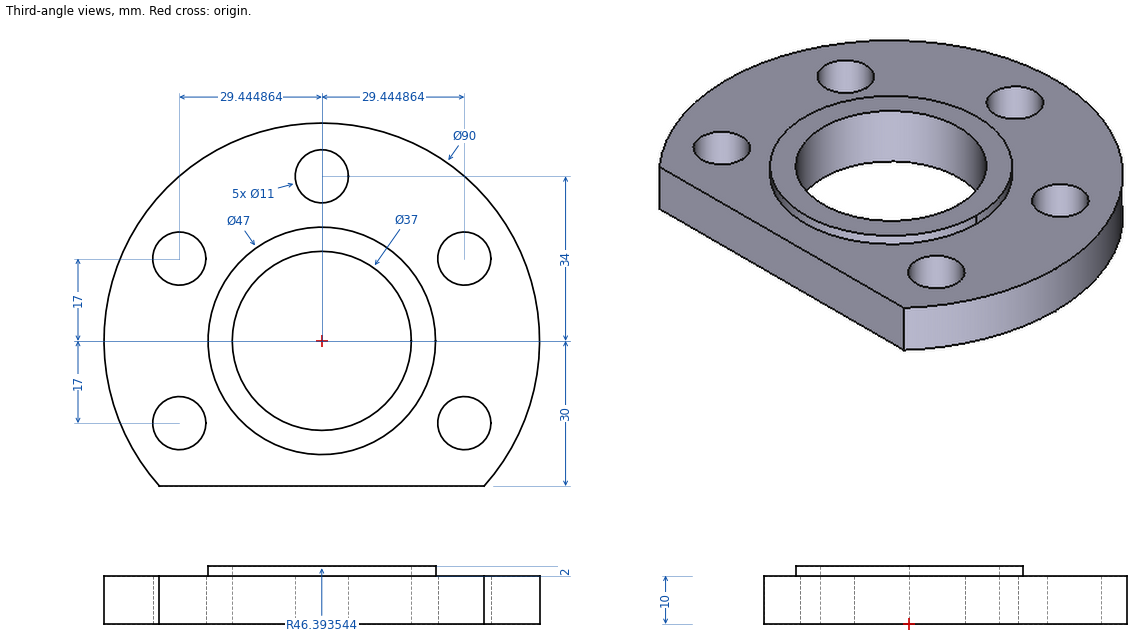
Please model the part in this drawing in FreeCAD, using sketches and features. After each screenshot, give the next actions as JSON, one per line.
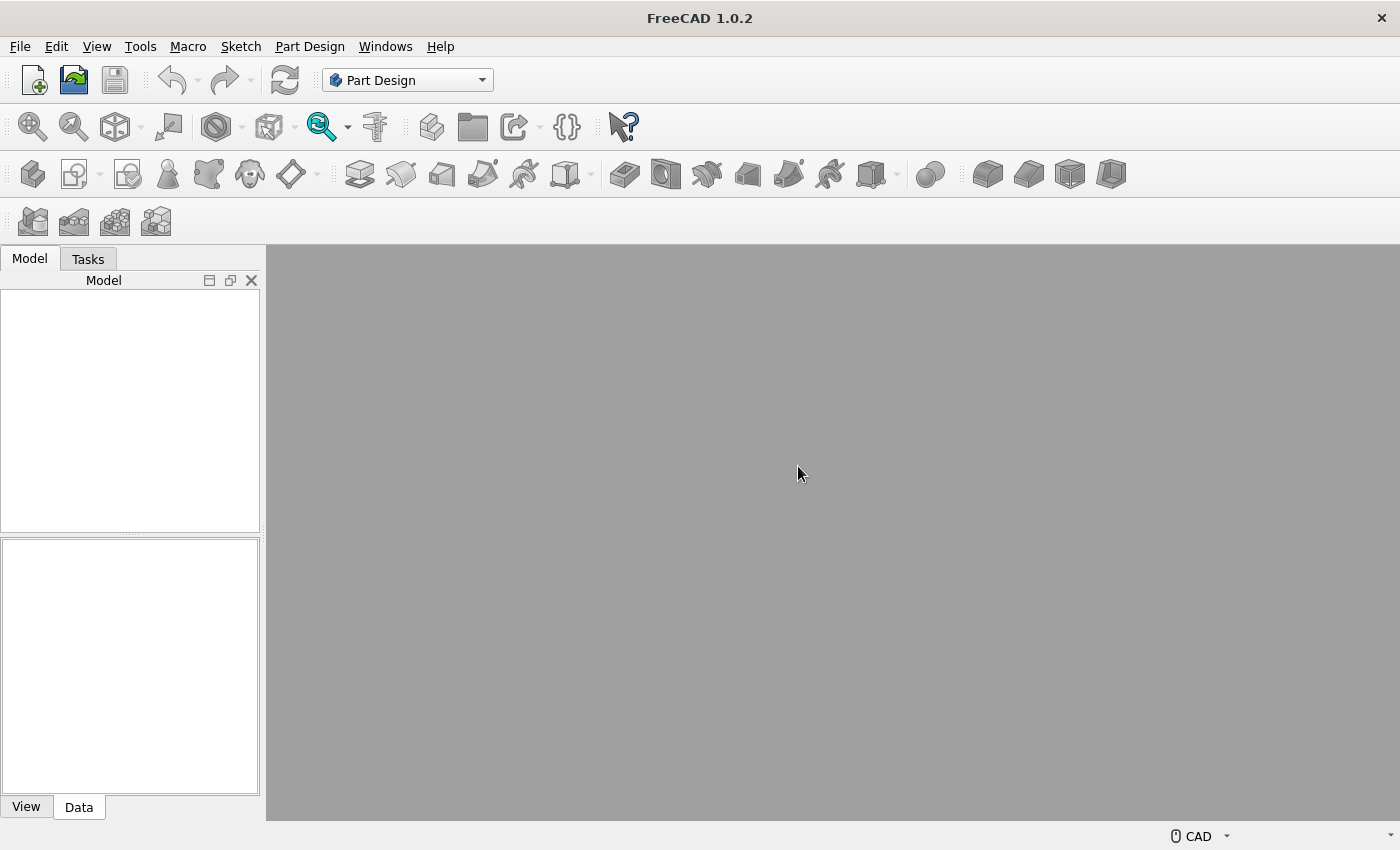
{"action": "left_click", "coordinate": [33, 80]}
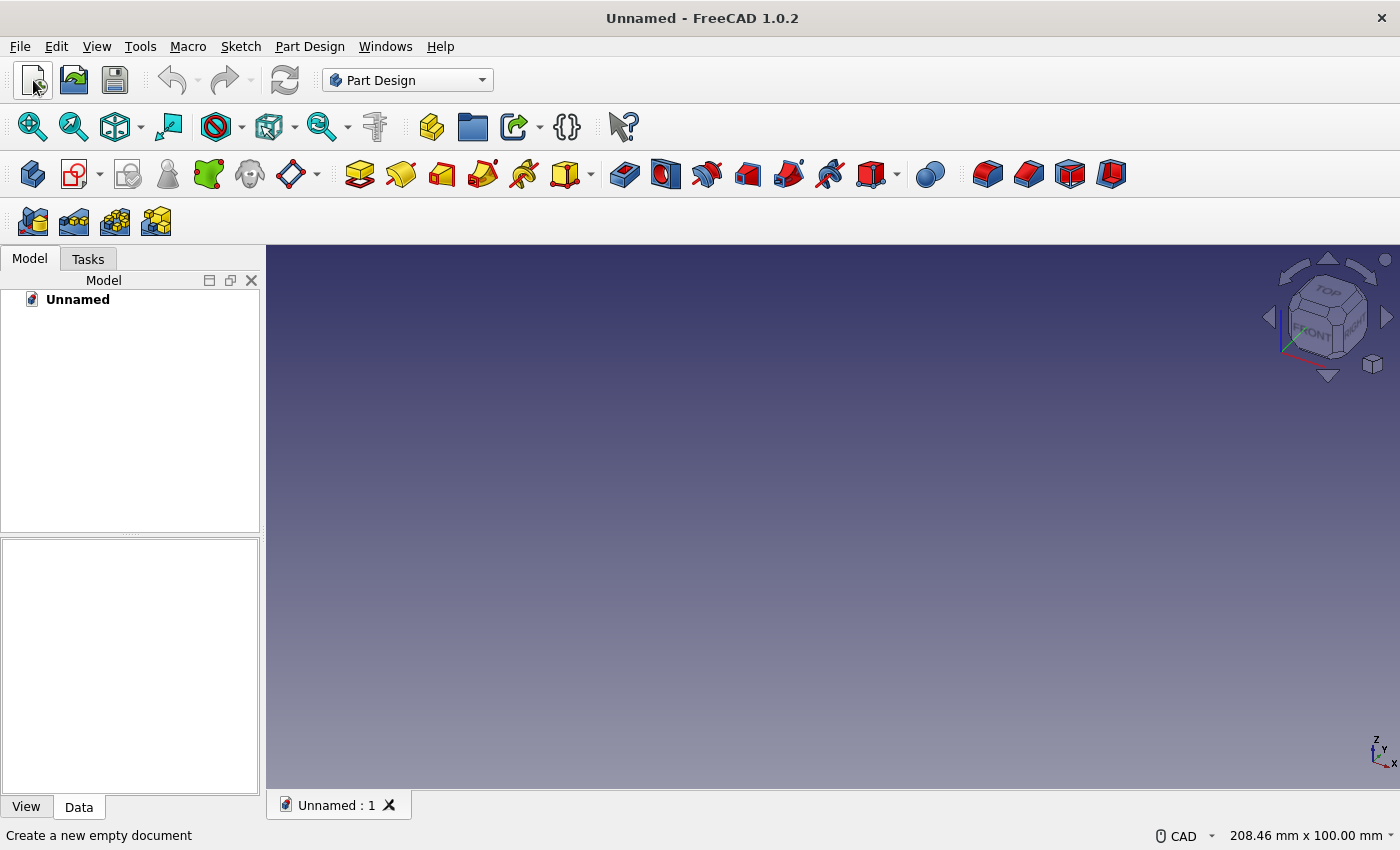
{"action": "left_click", "coordinate": [74, 174]}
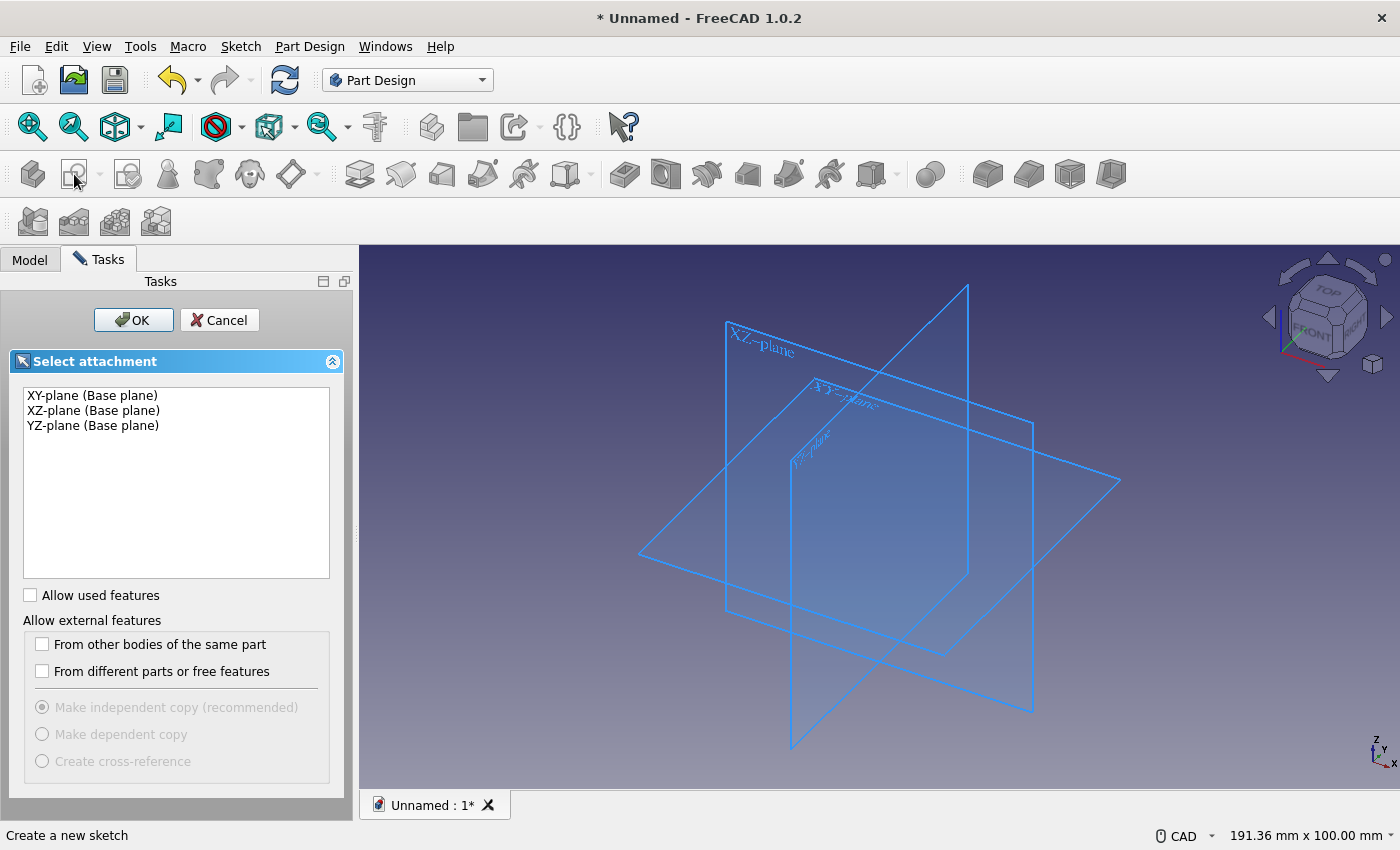
{"action": "left_click", "coordinate": [84, 396]}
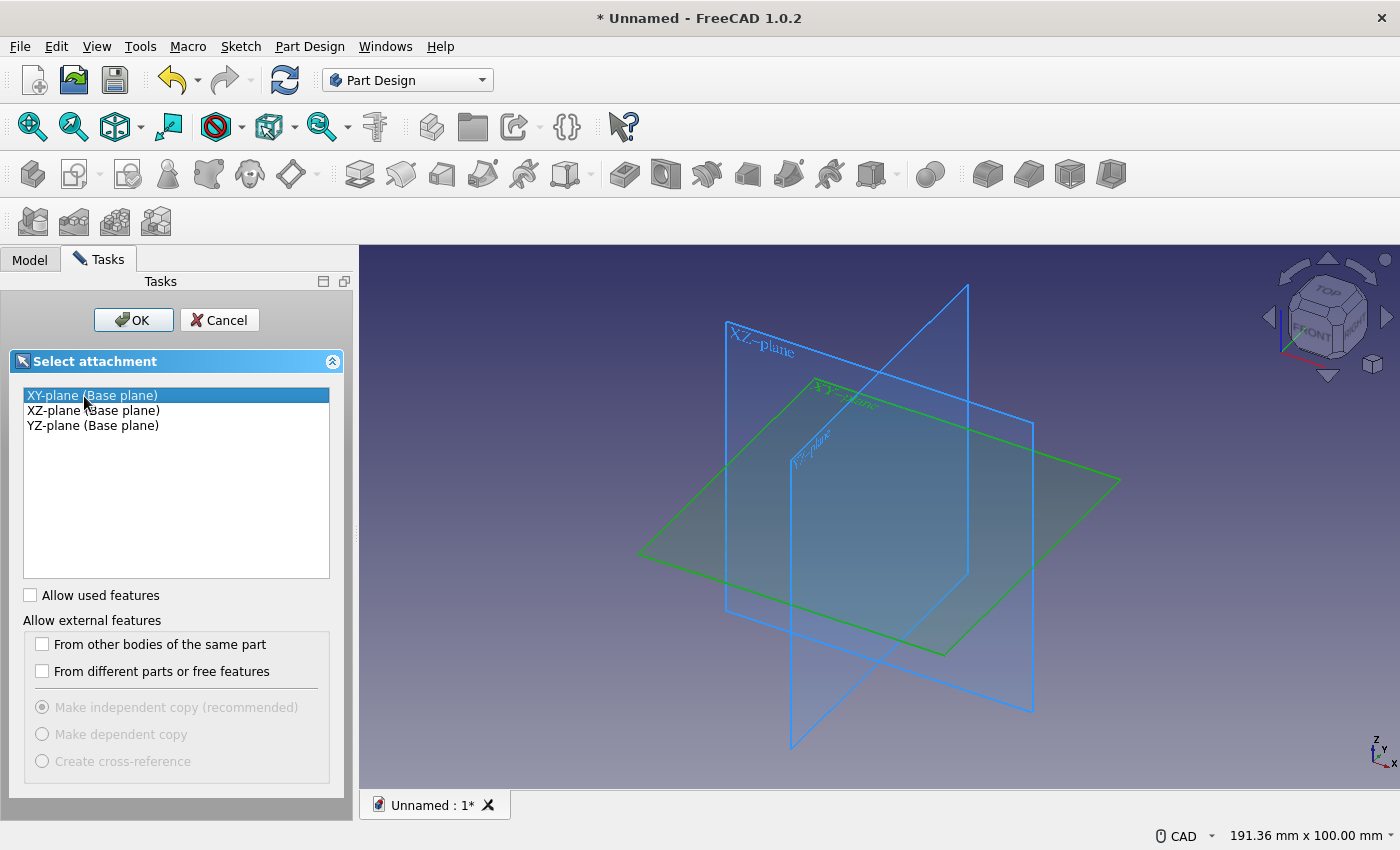
{"action": "left_click", "coordinate": [134, 320]}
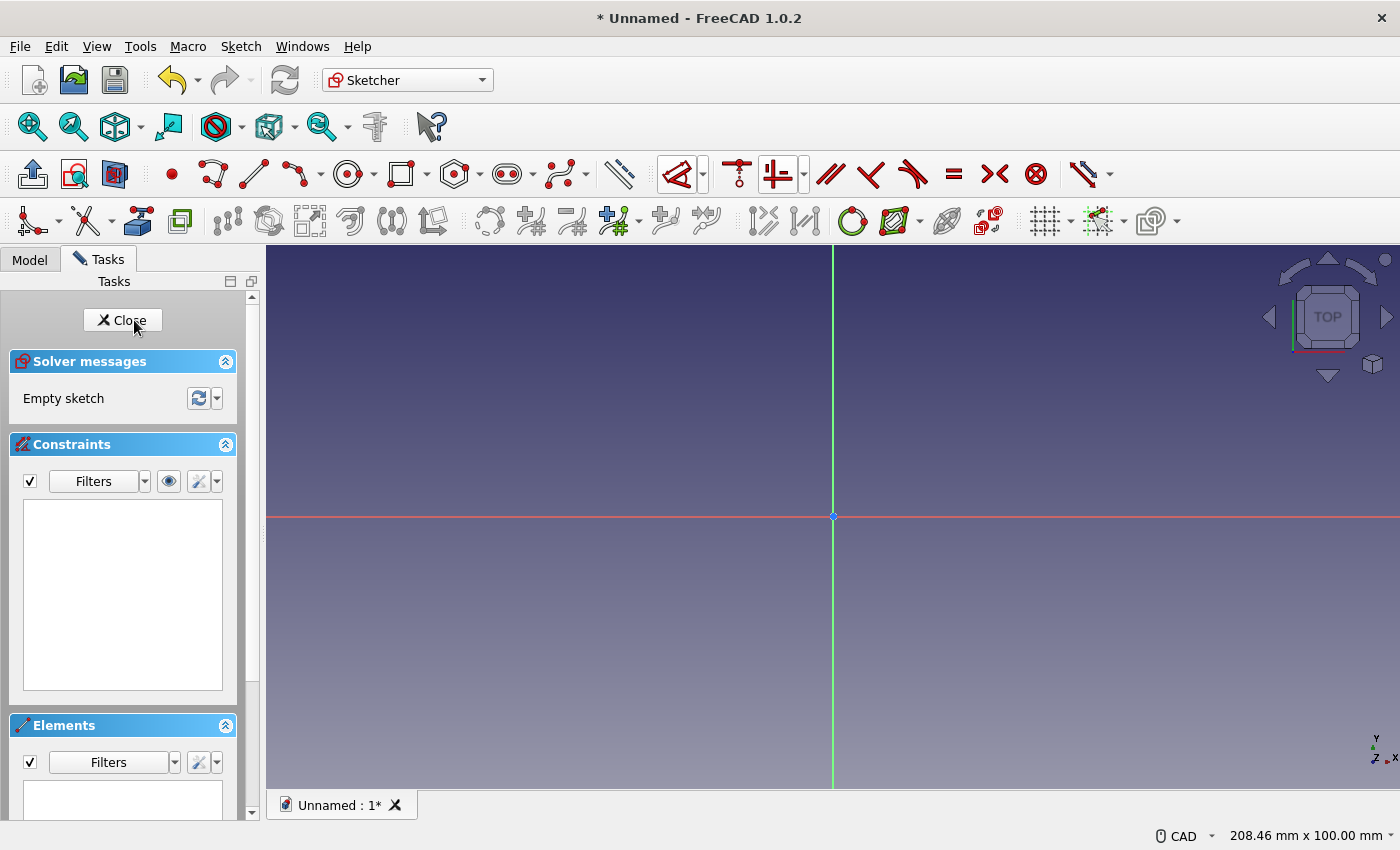
{"action": "scroll", "coordinate": [625, 517], "scroll_direction": "down", "scroll_amount": 2}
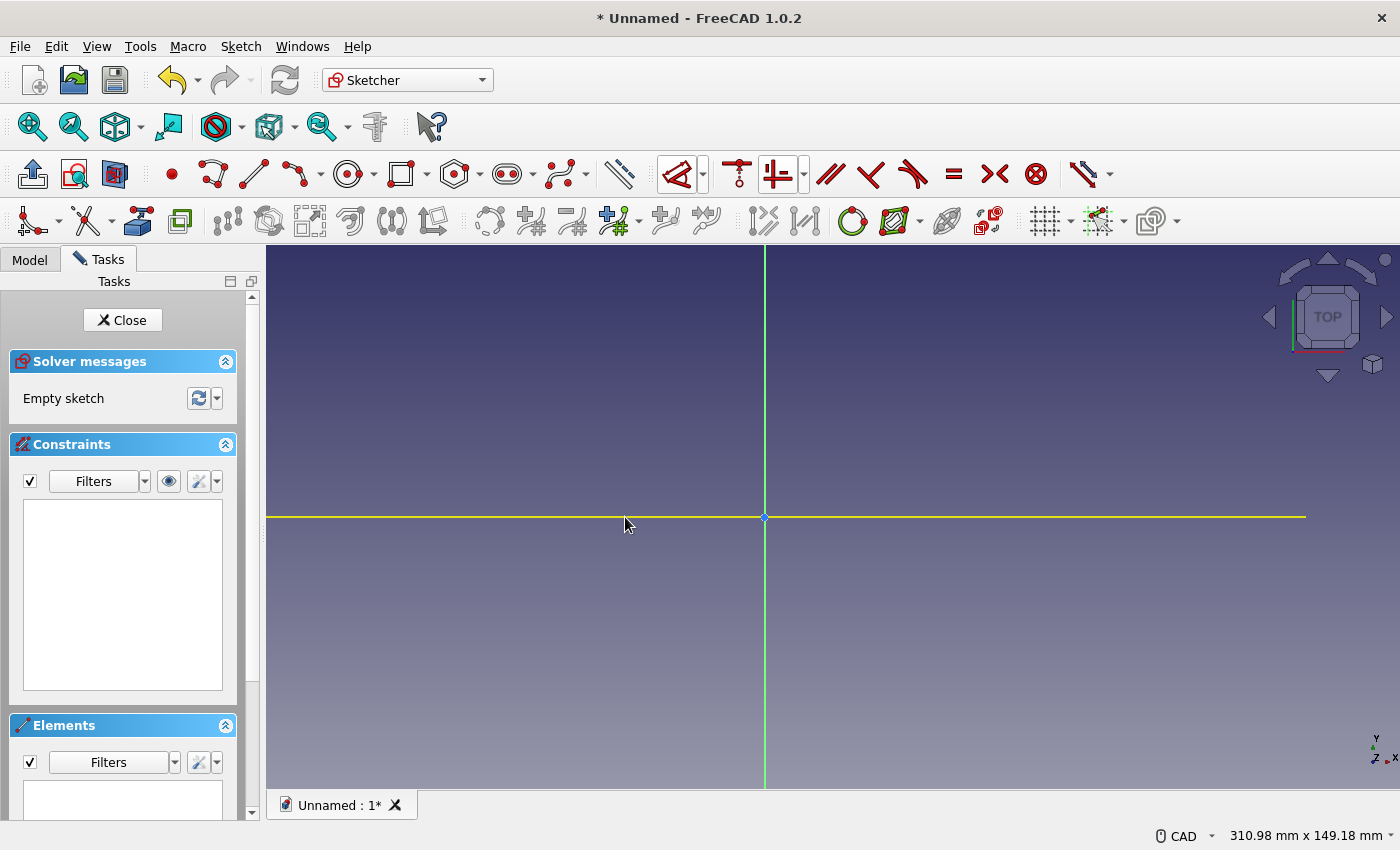
{"action": "left_click", "coordinate": [348, 174]}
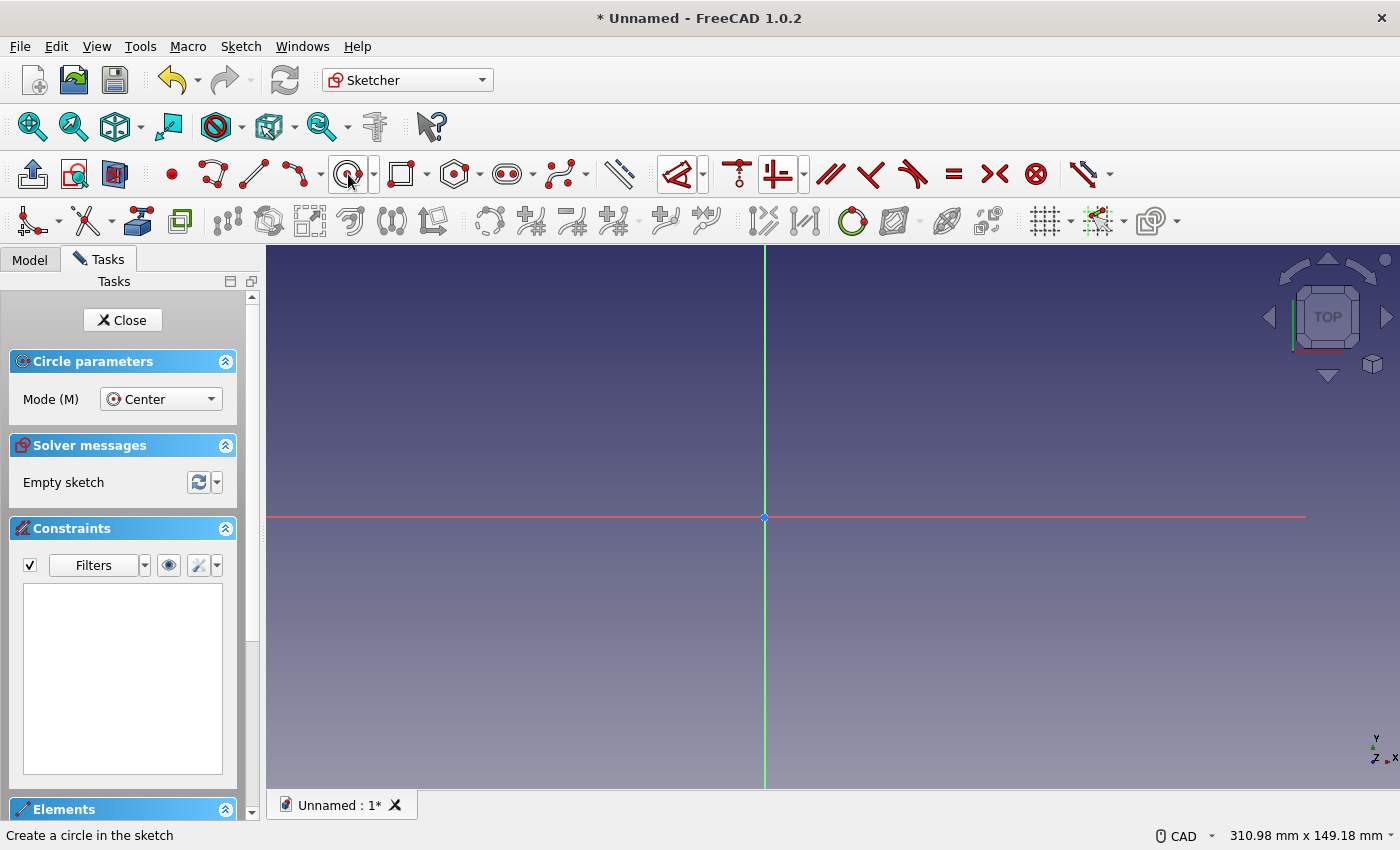
{"action": "left_click", "coordinate": [765, 517]}
{"action": "left_click", "coordinate": [881, 401]}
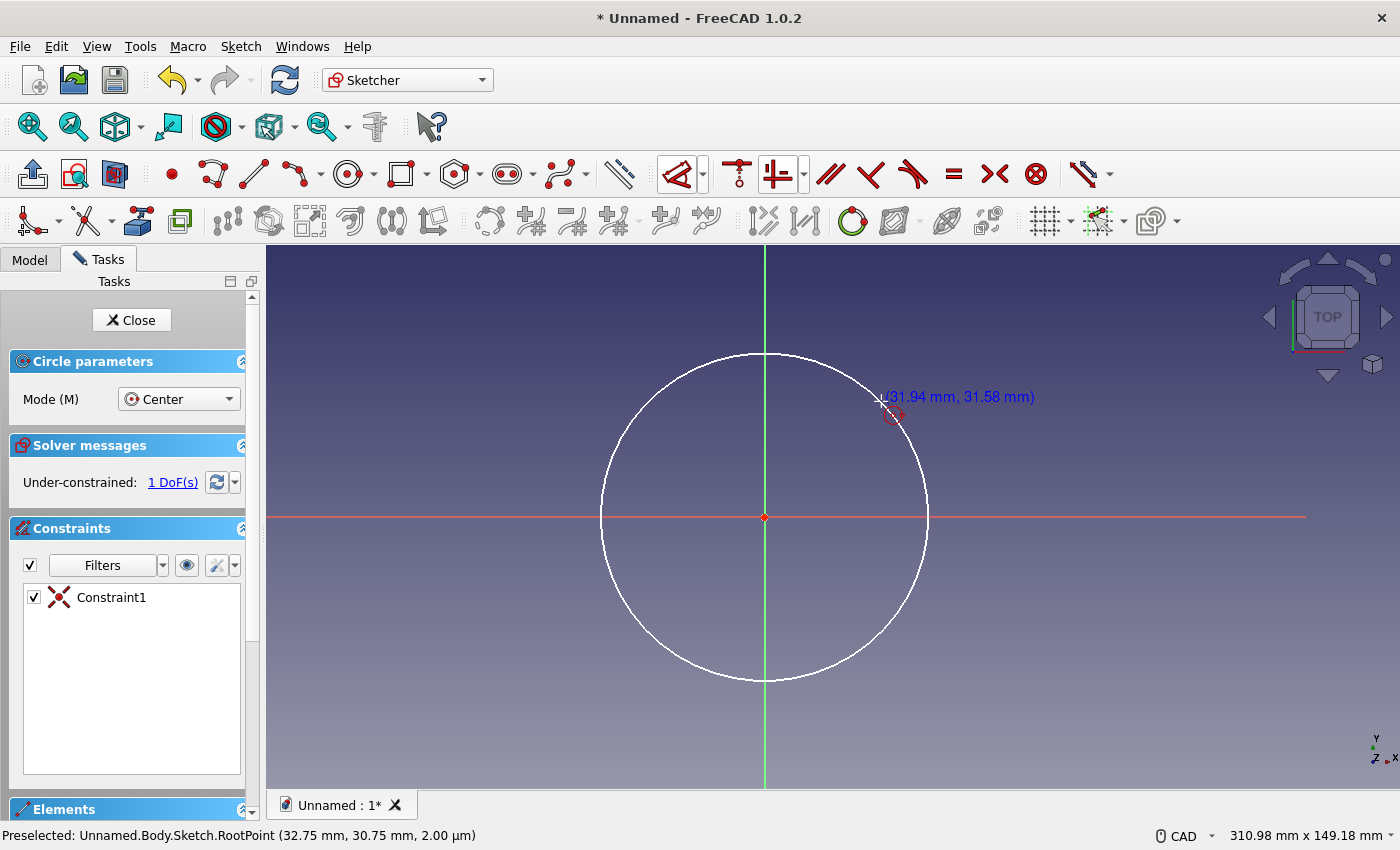
{"action": "left_click", "coordinate": [765, 517]}
{"action": "left_click", "coordinate": [812, 469]}
{"action": "key", "text": "Escape"}